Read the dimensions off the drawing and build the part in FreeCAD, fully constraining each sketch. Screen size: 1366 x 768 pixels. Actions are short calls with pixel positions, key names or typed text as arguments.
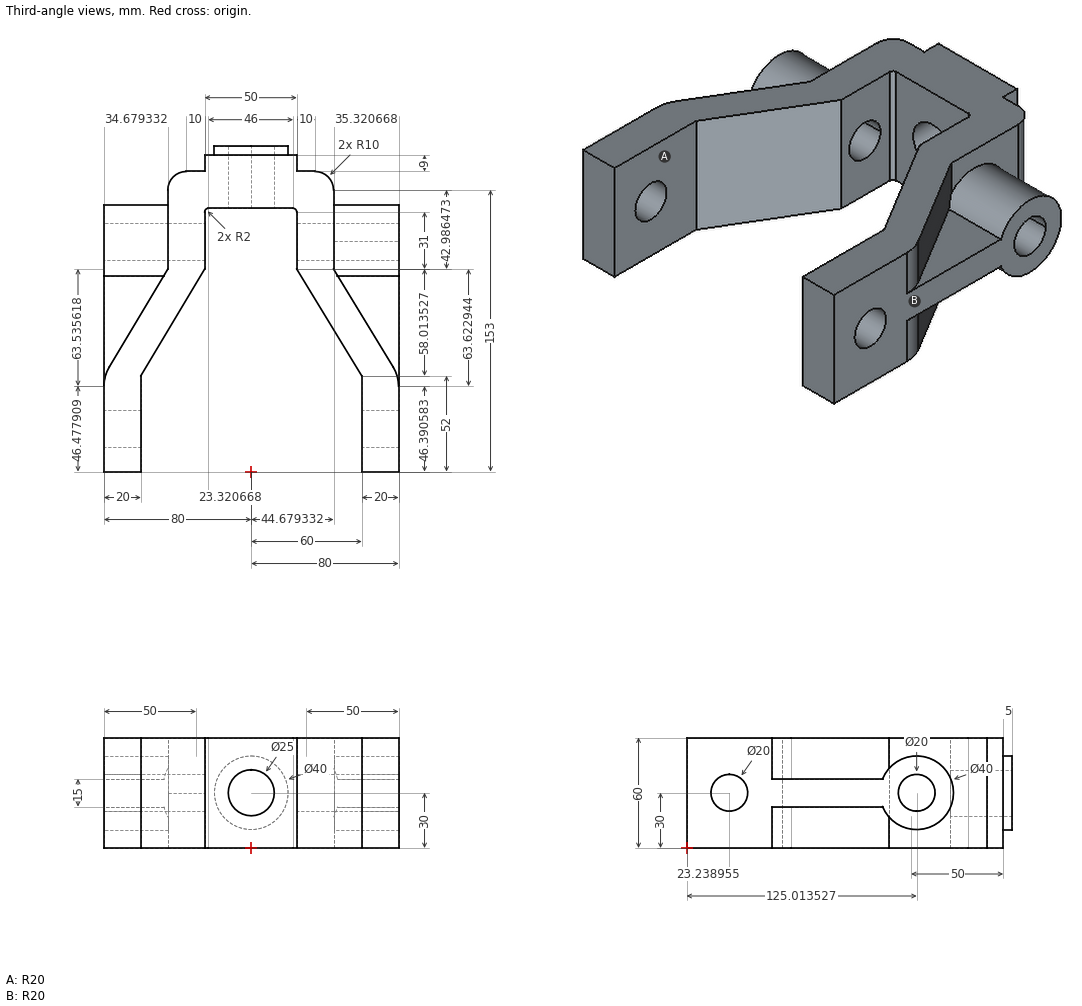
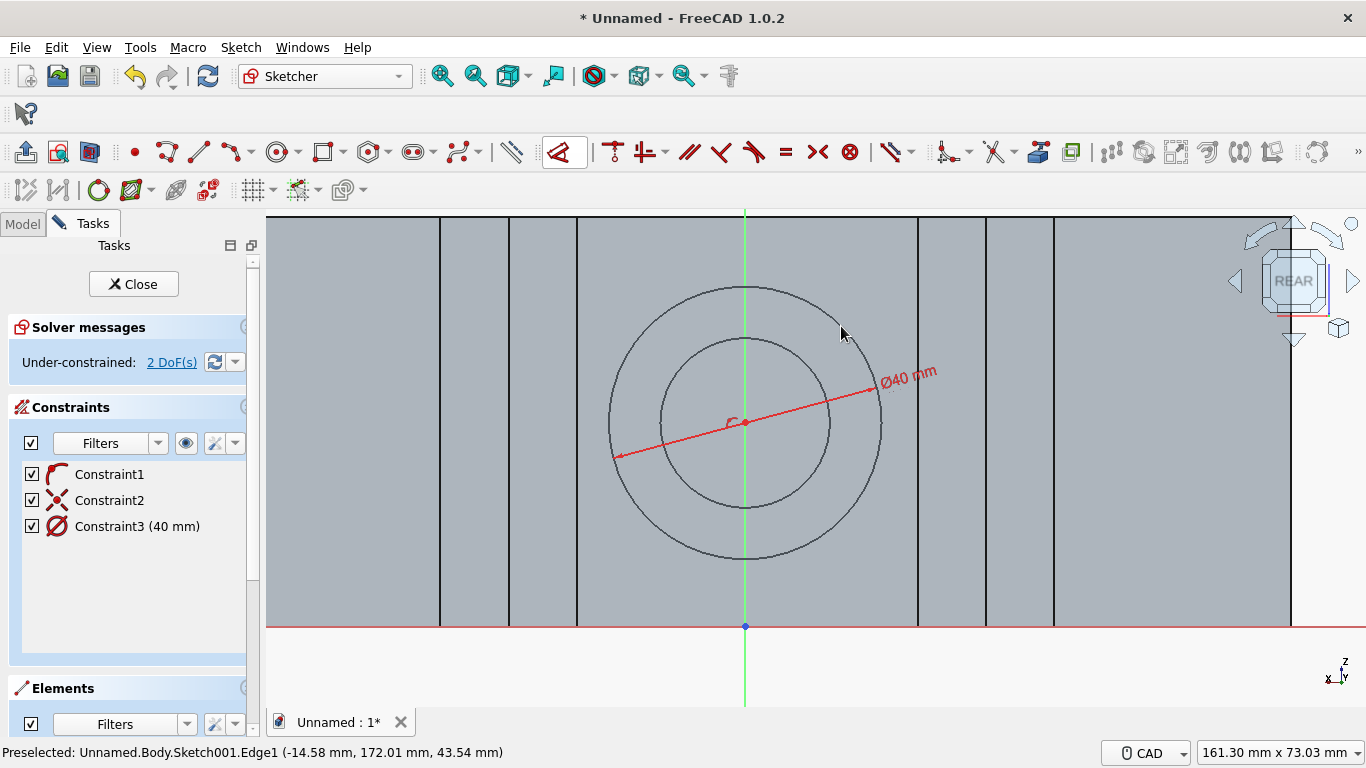
click(805, 363)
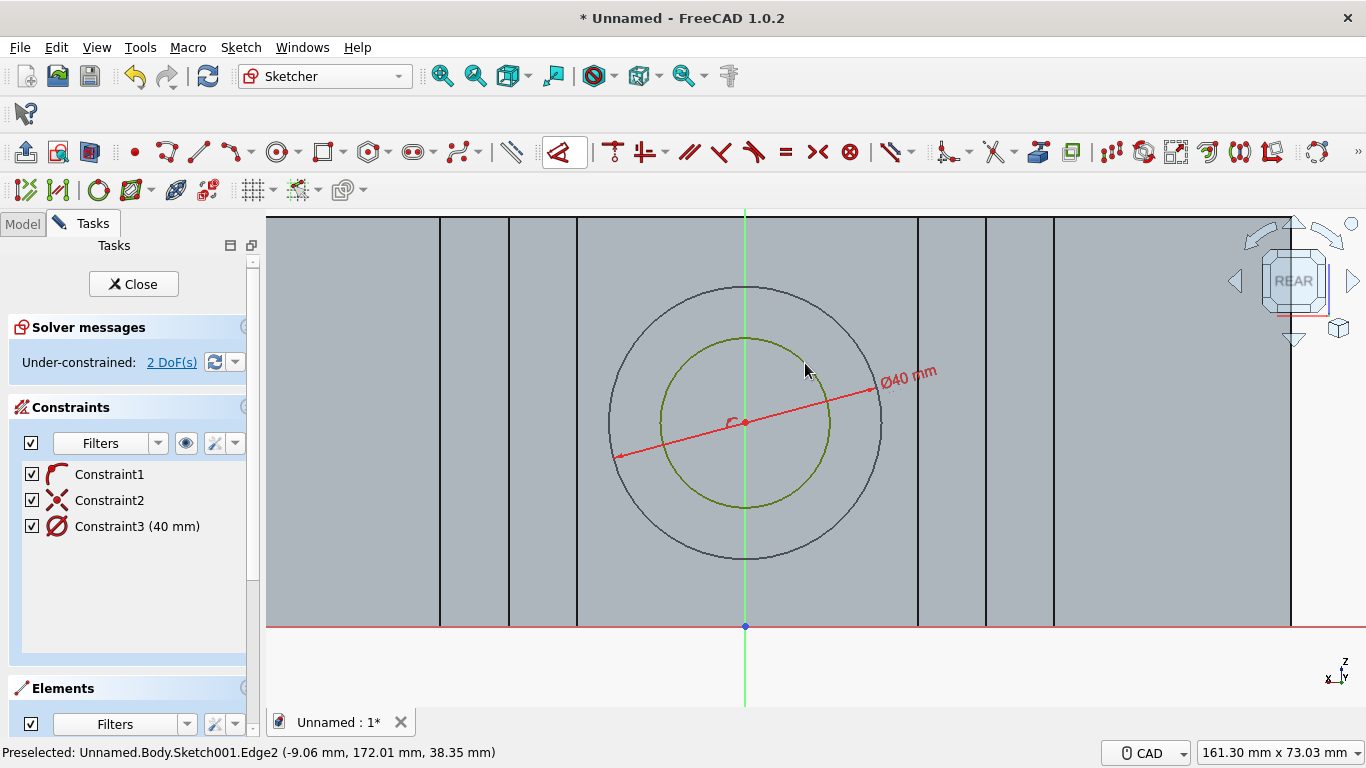
key(k)
key(o)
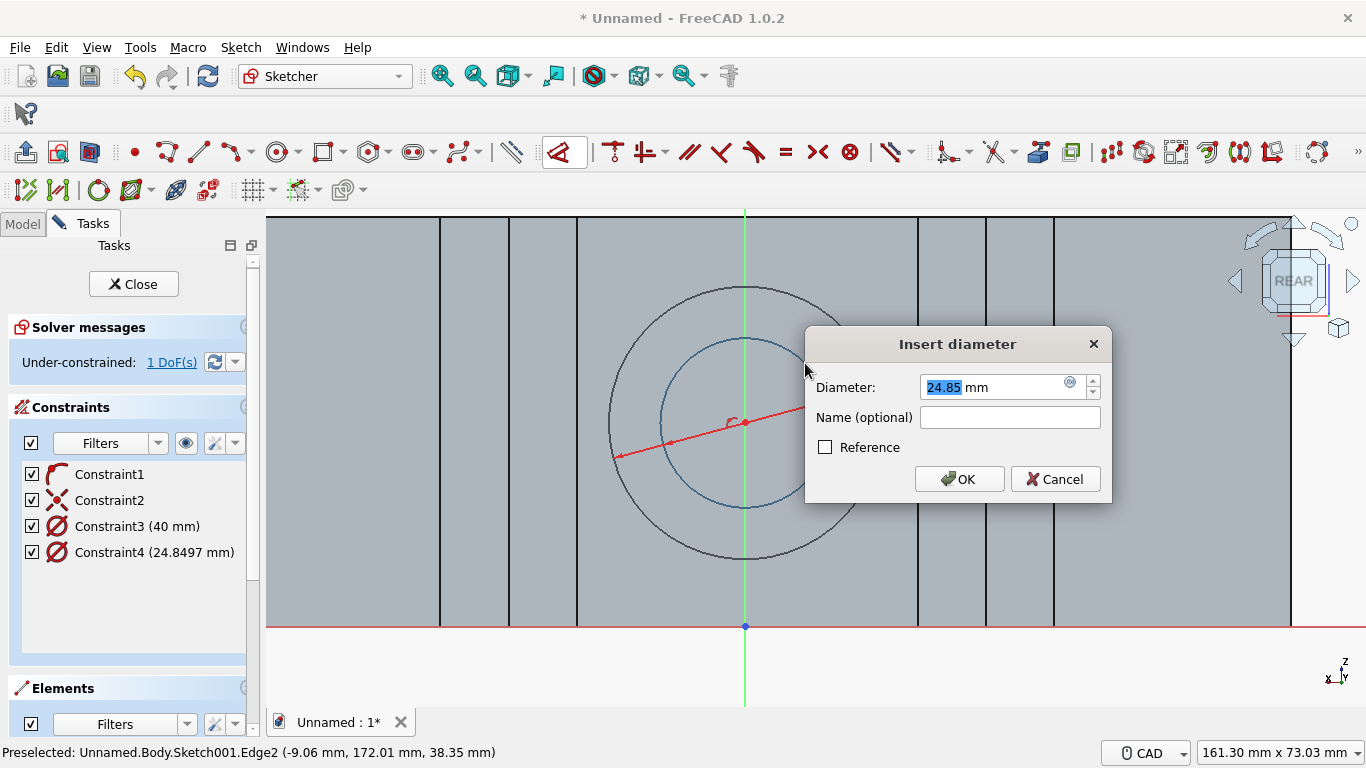
text(25)
key(Return)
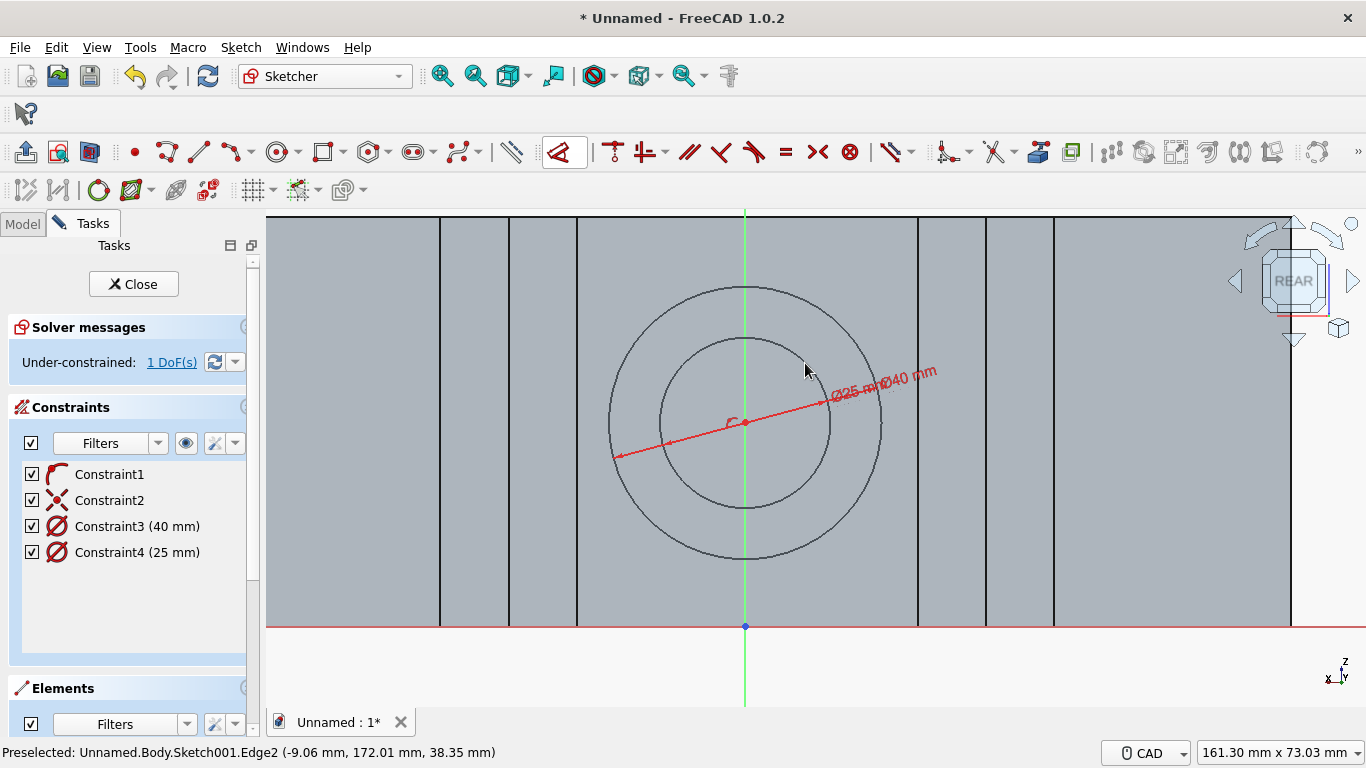
click(745, 423)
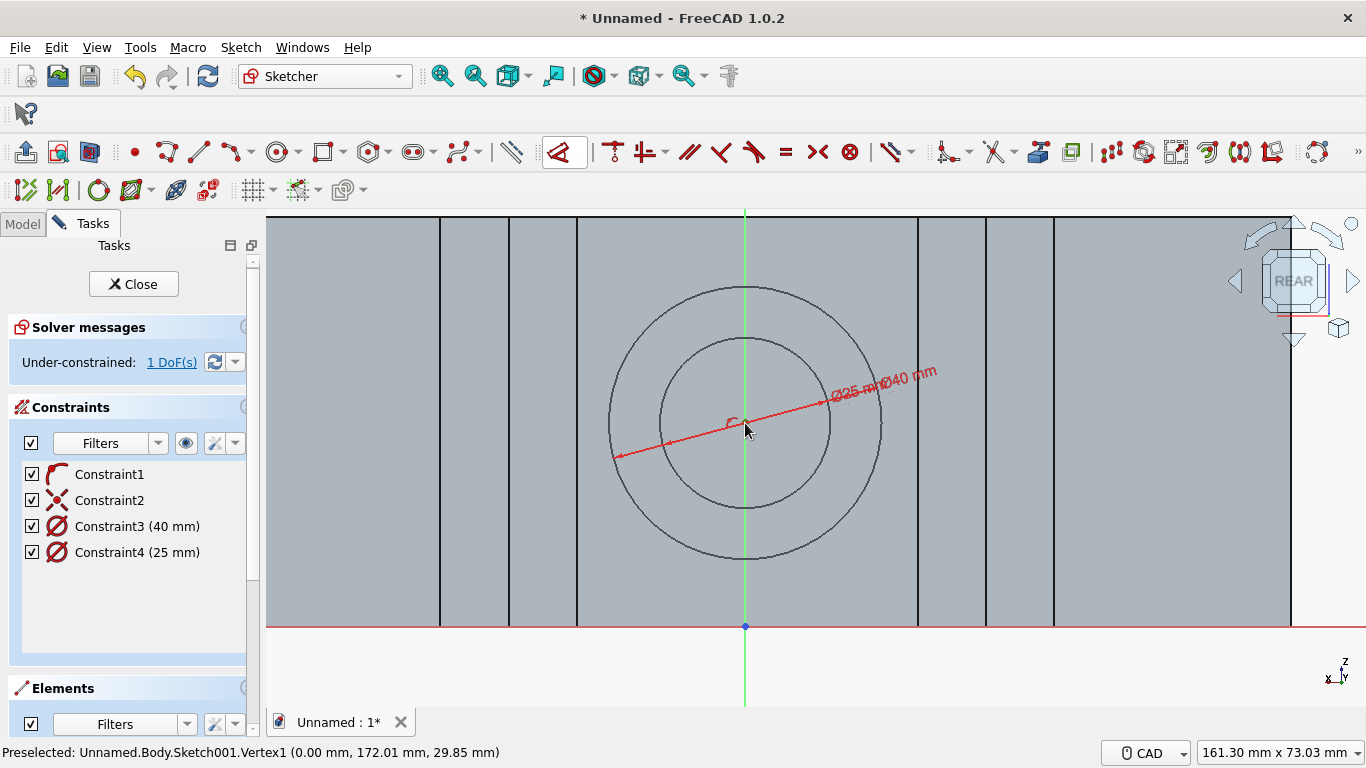
key(i)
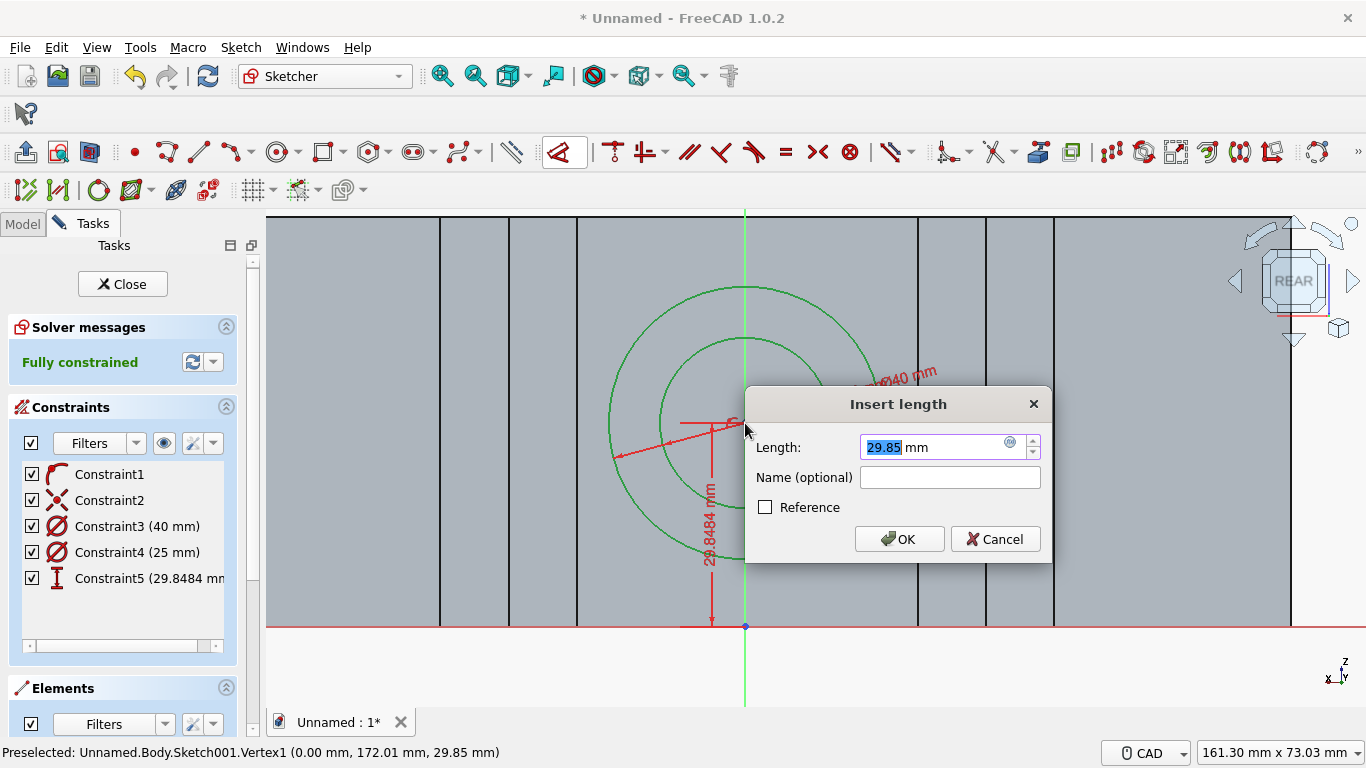
text(30)
key(Return)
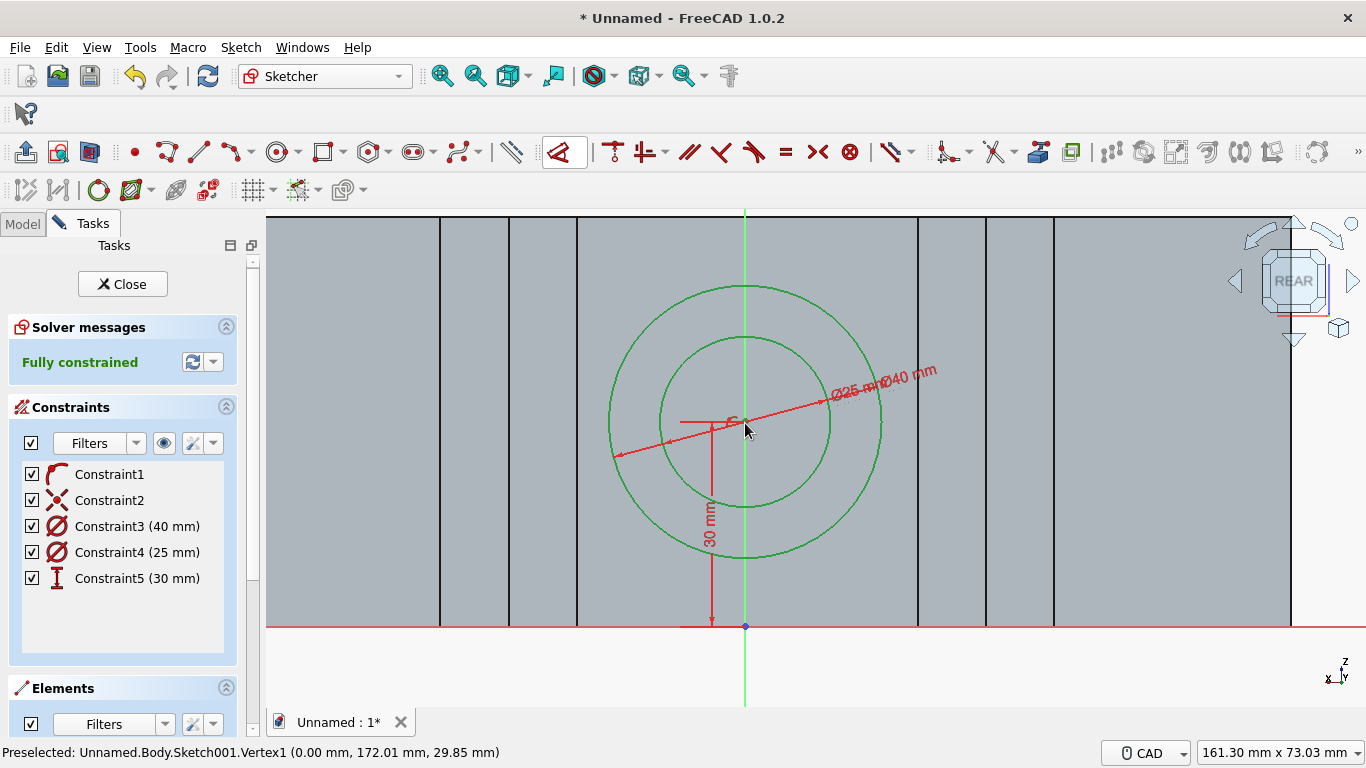
click(123, 284)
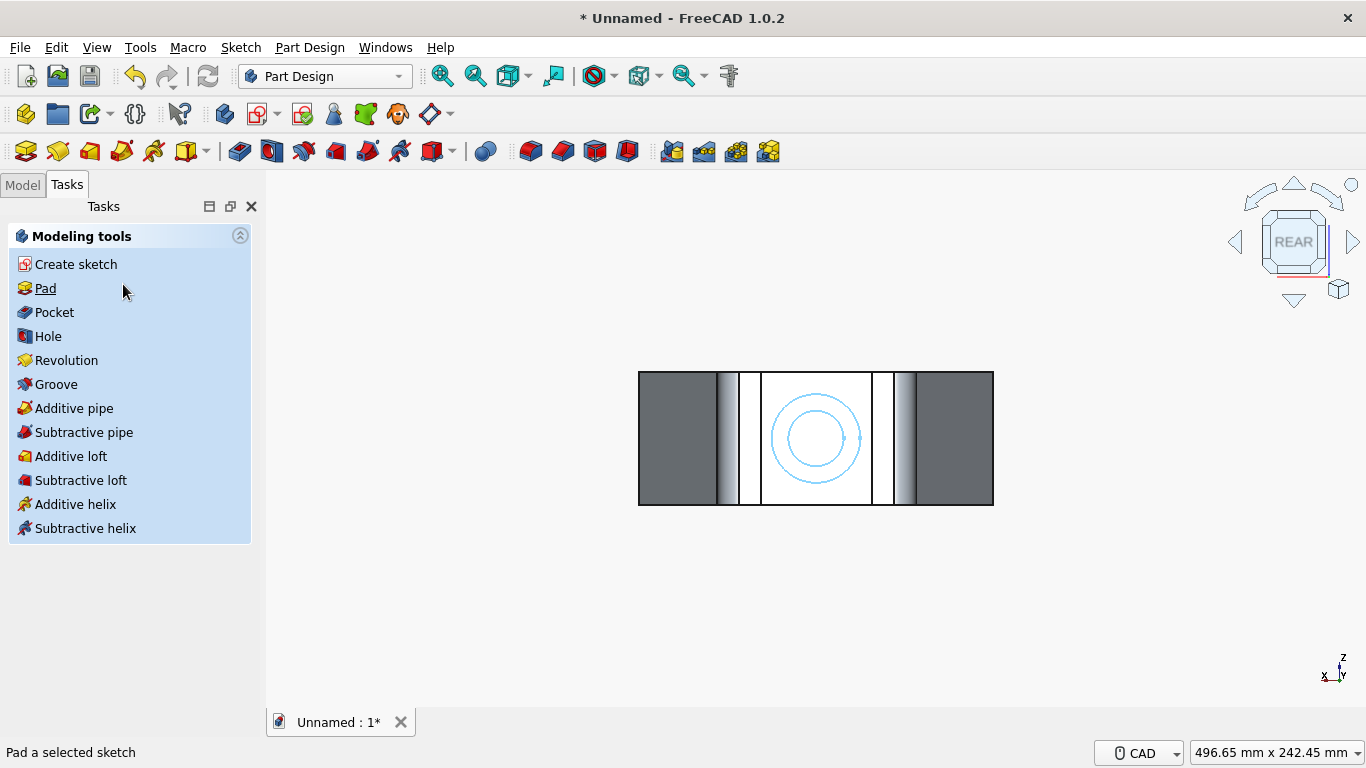
click(26, 152)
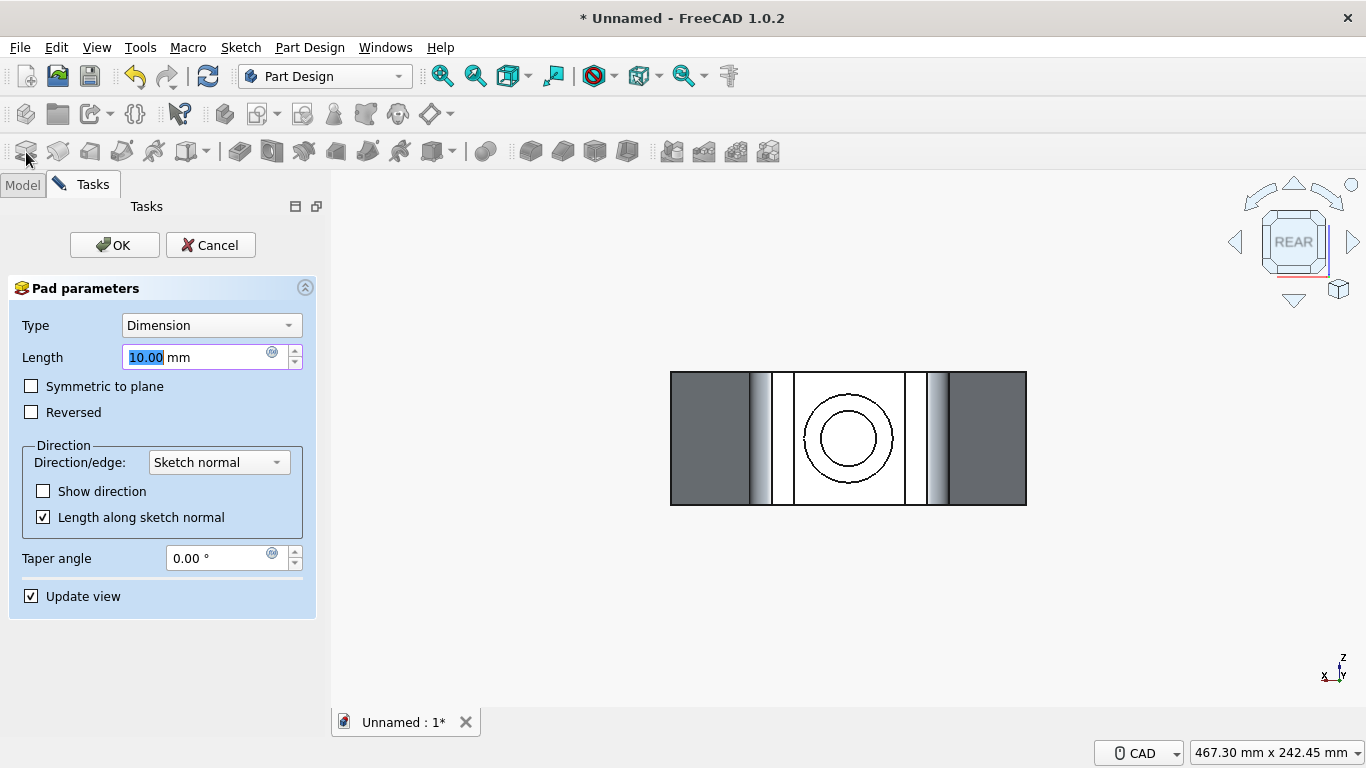
text(5)
key(Tab)